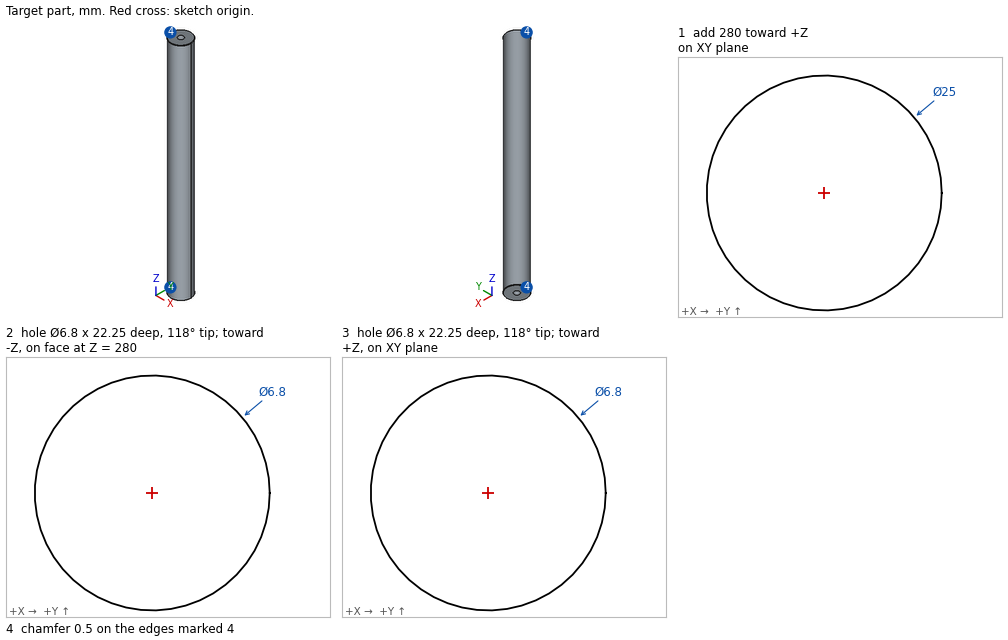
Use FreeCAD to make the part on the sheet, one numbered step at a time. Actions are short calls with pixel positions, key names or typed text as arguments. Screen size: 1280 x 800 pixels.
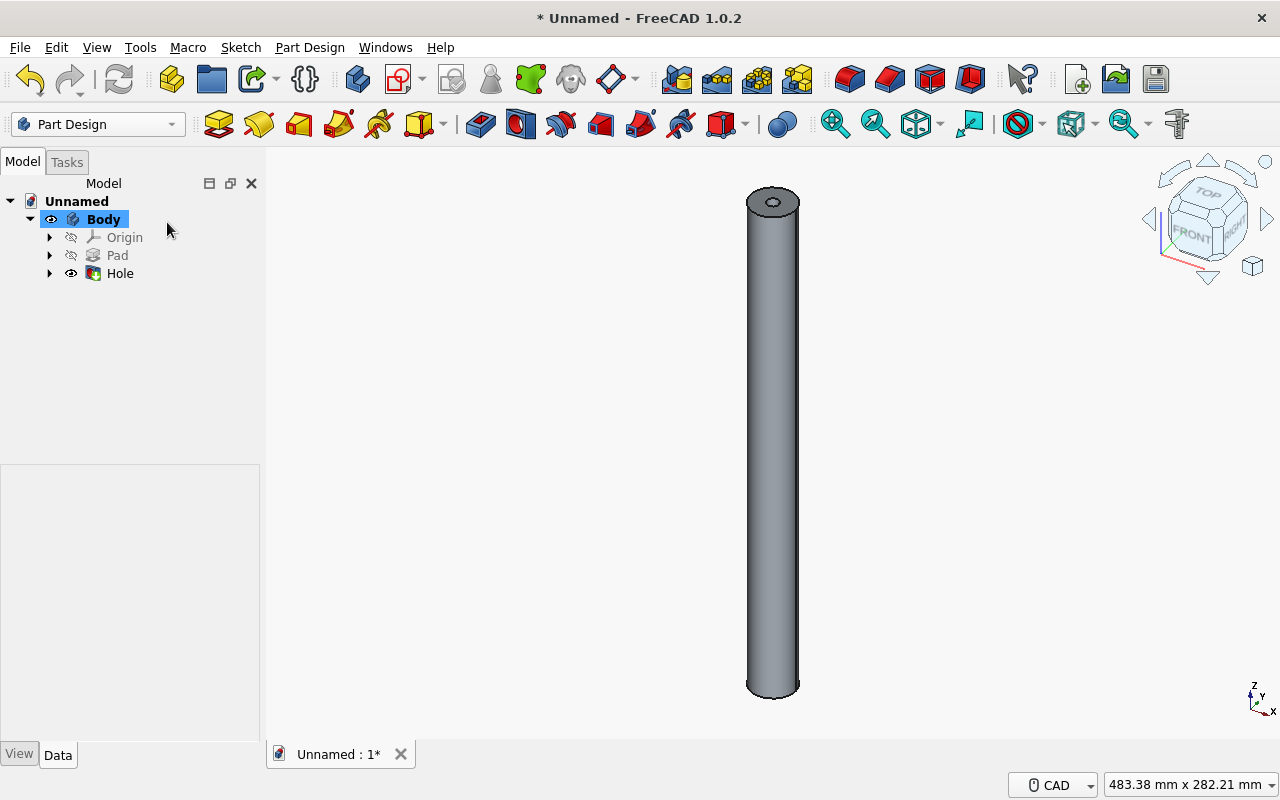
click(398, 80)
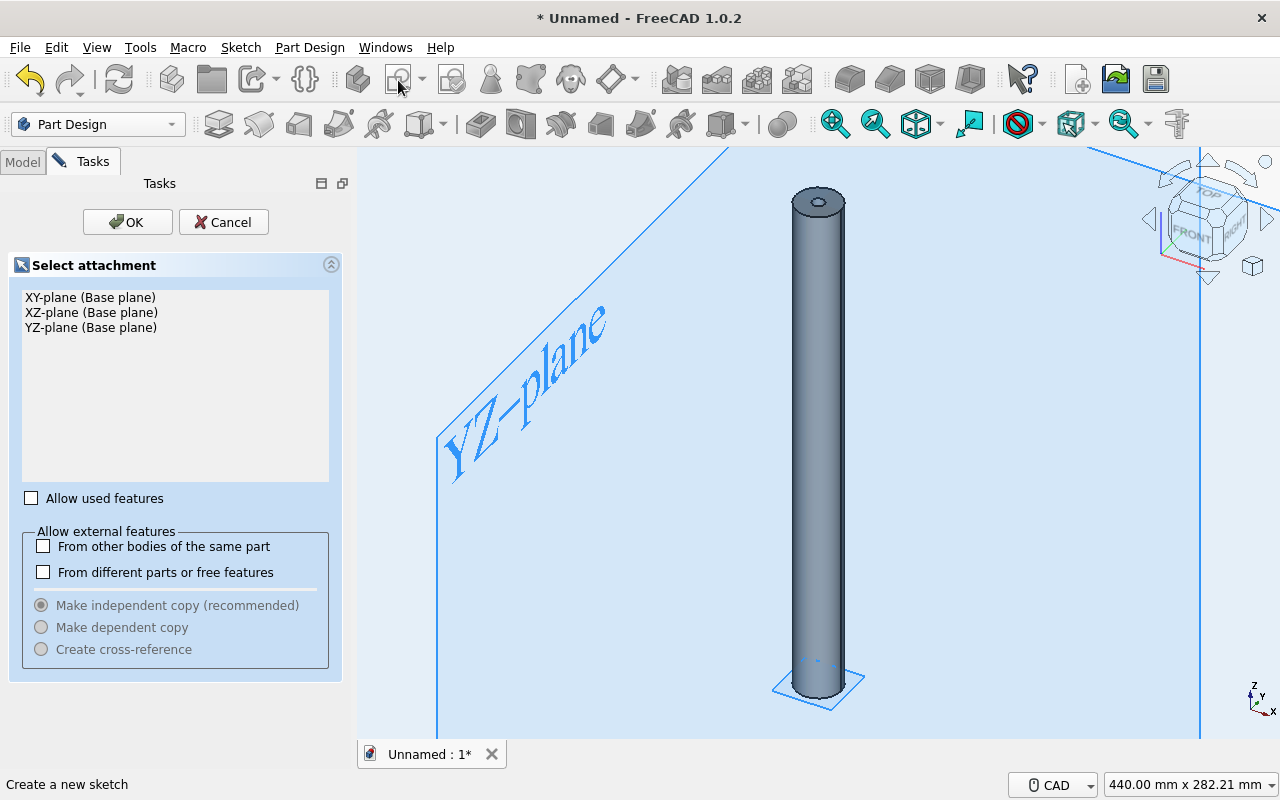
click(82, 298)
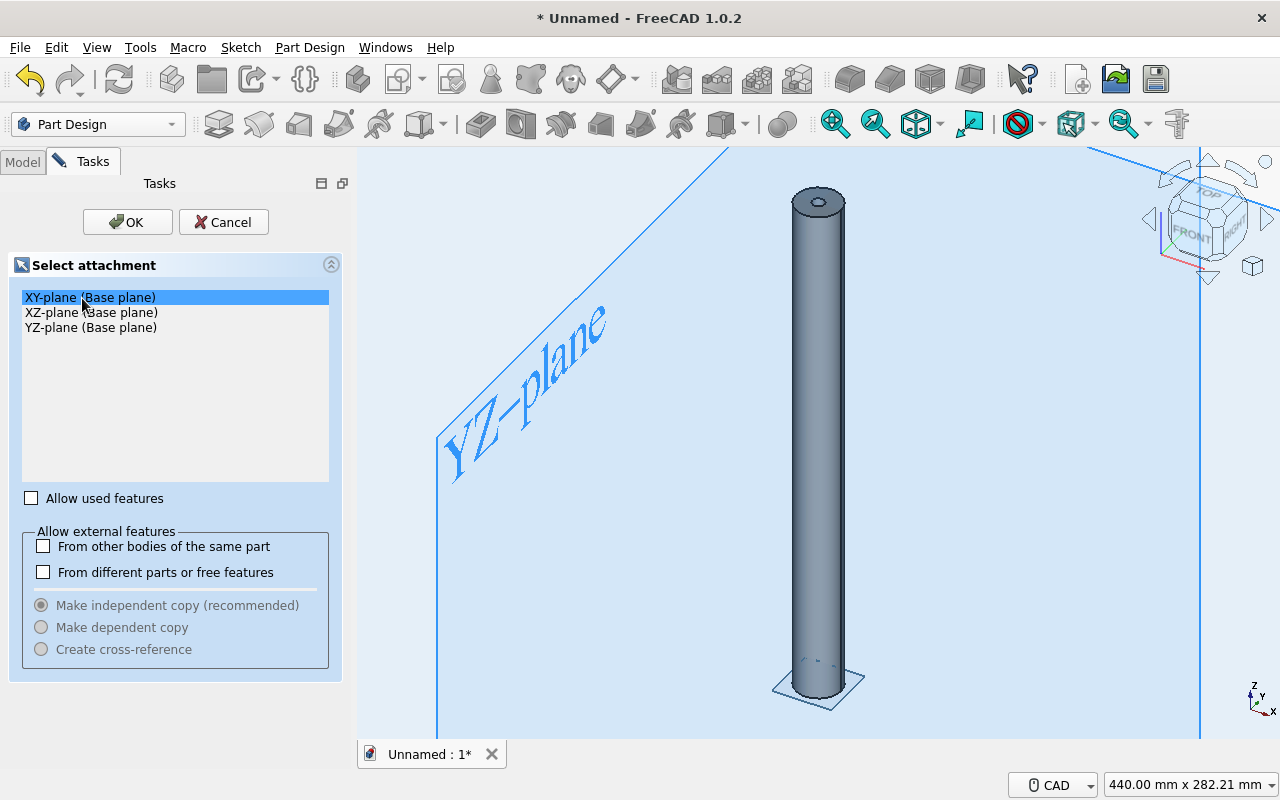
click(128, 222)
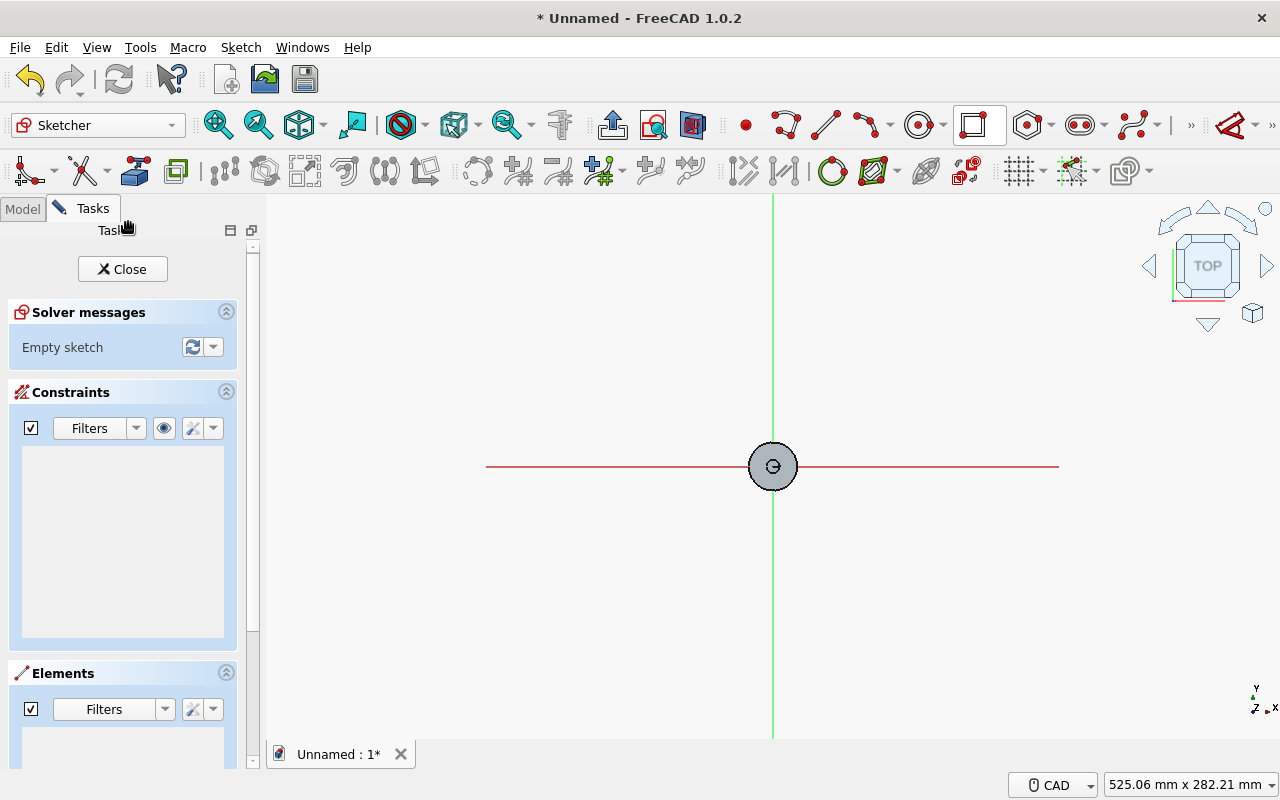
click(694, 126)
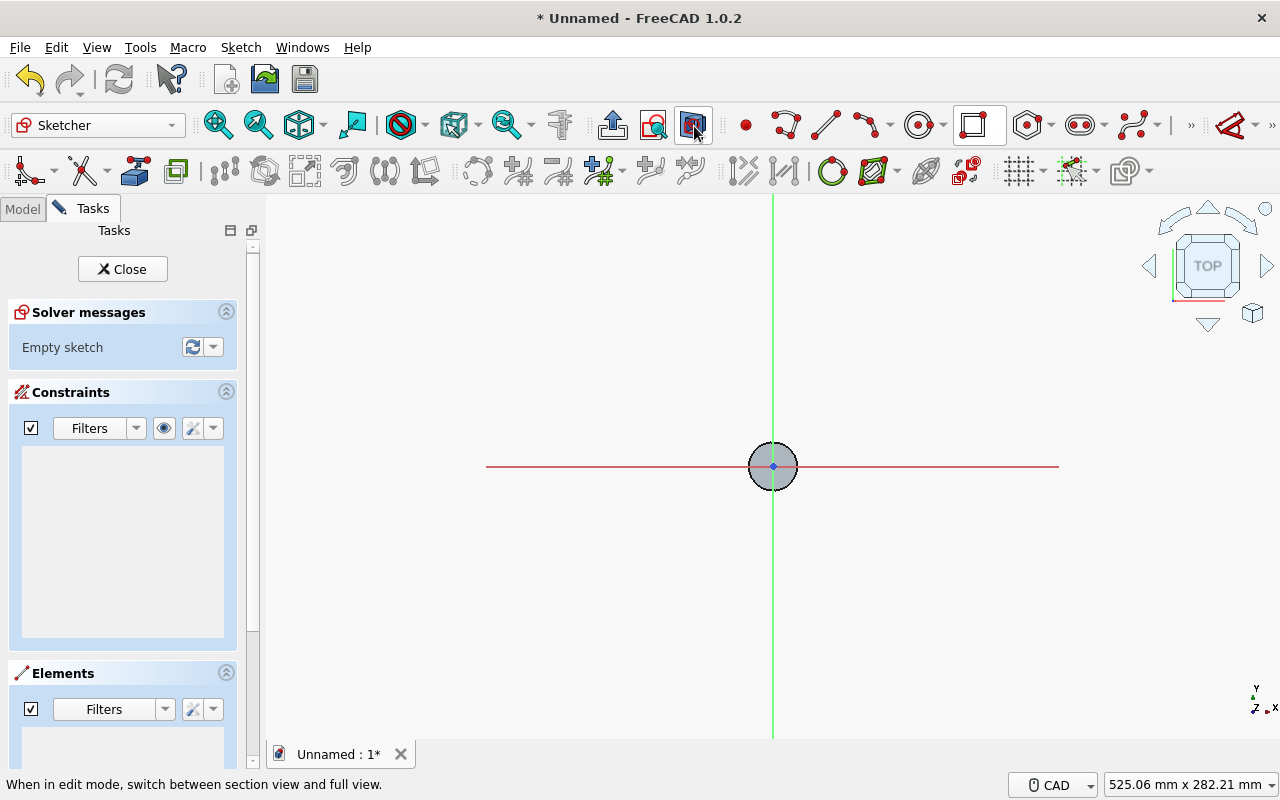
scroll(777, 466, up, 15)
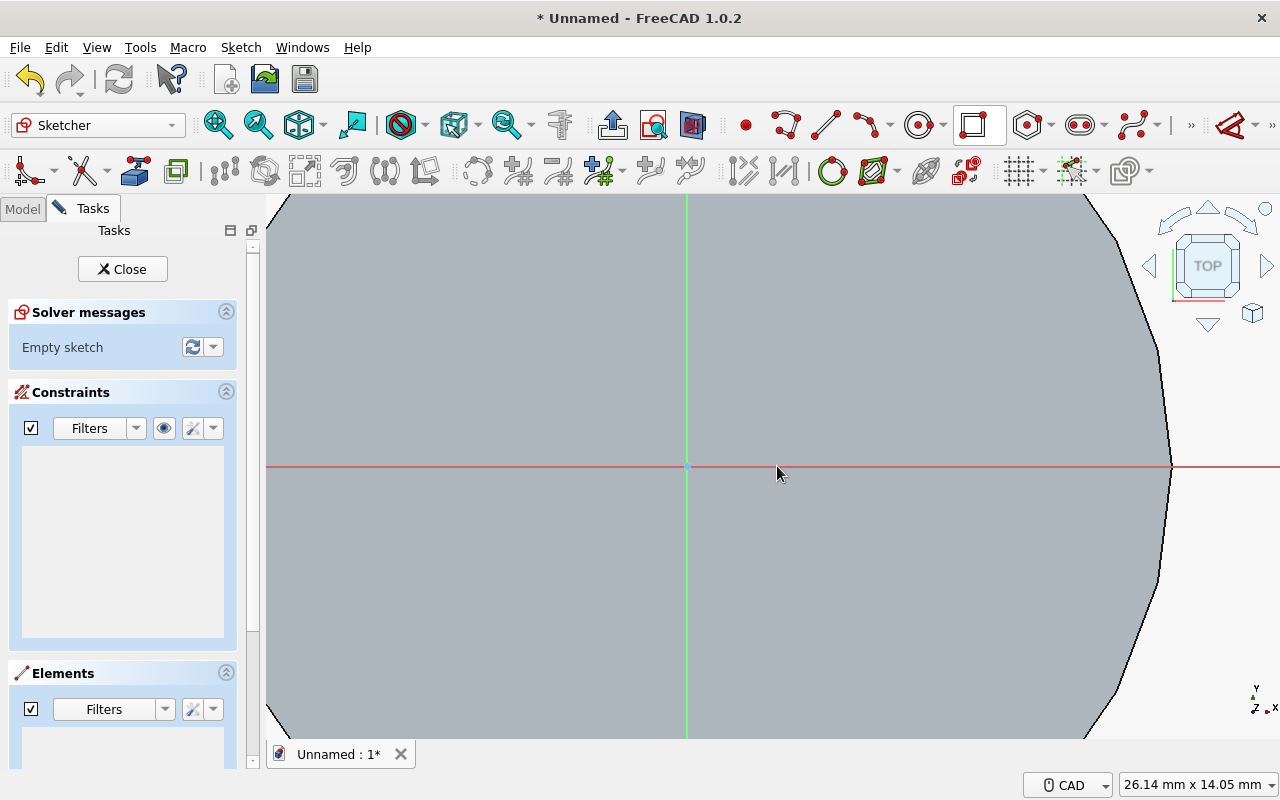
click(920, 126)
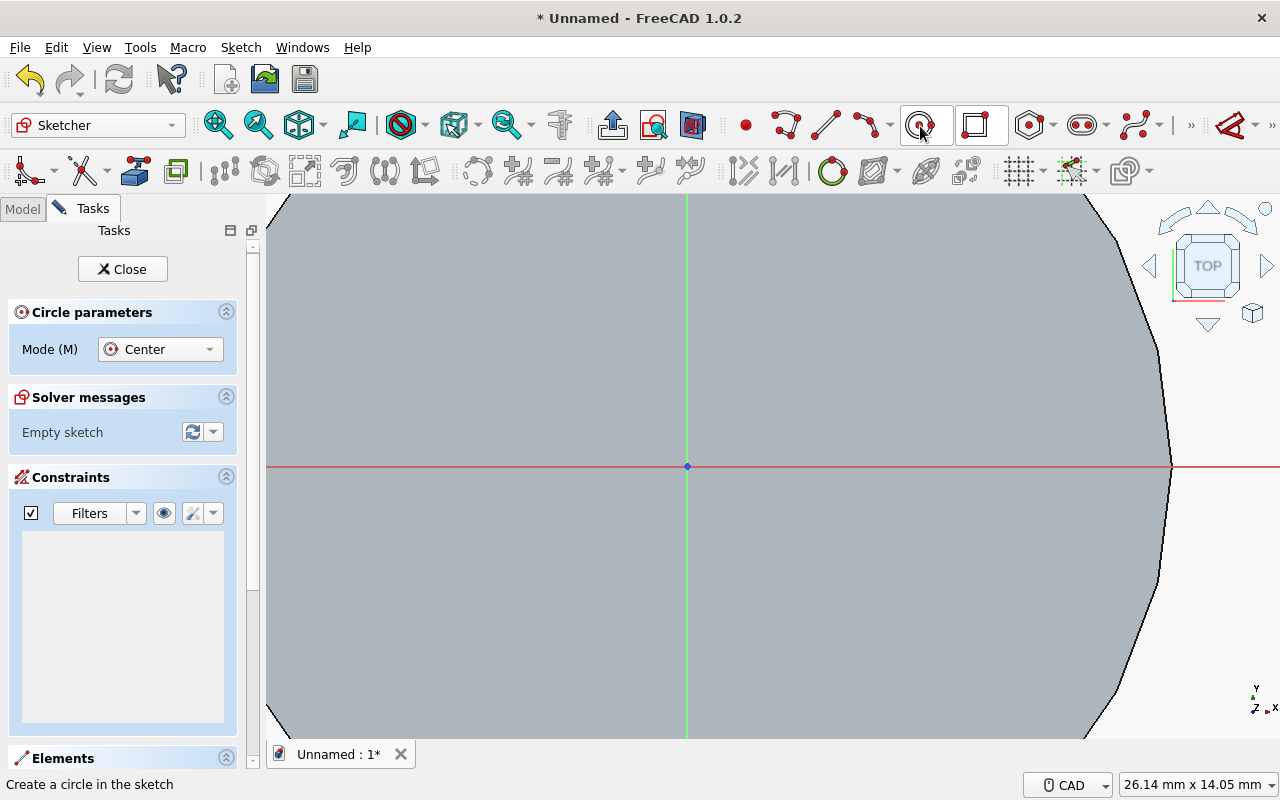
click(687, 466)
click(780, 373)
key(Escape)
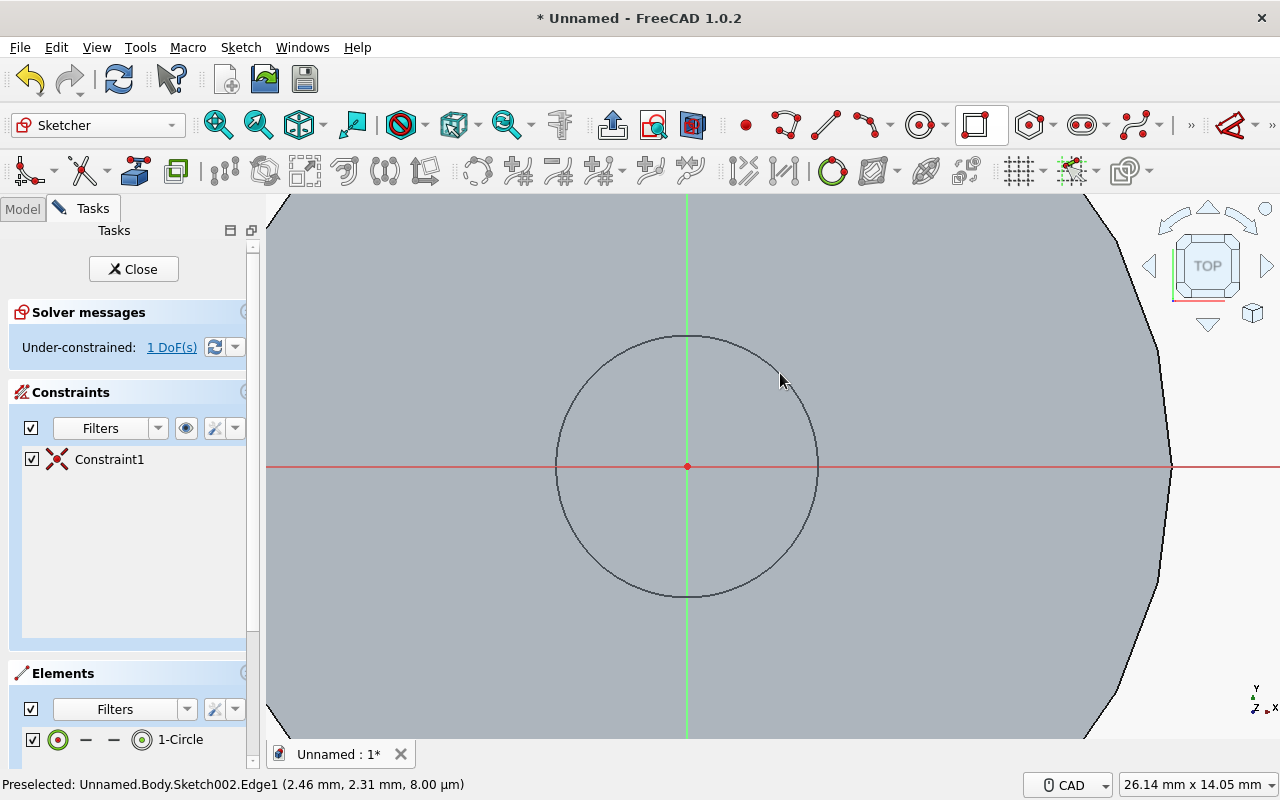
click(1230, 126)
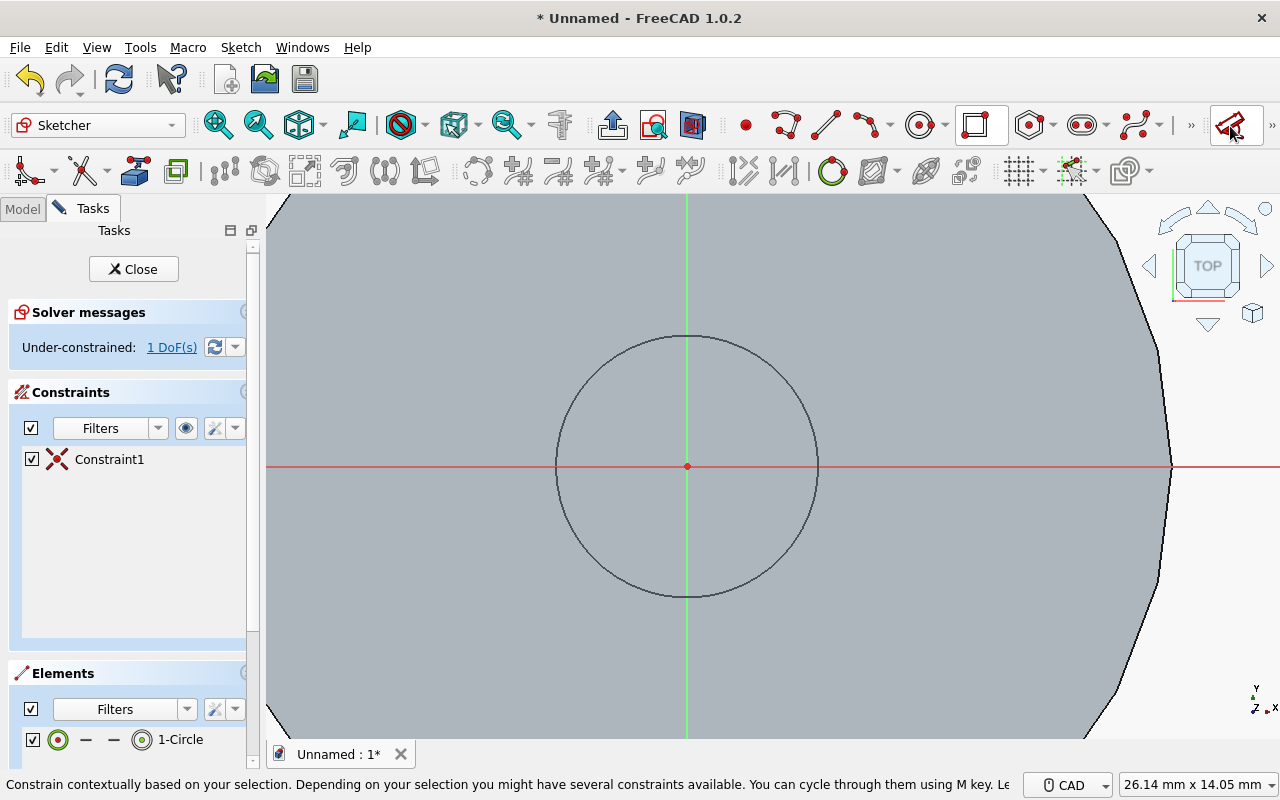
click(779, 373)
click(801, 350)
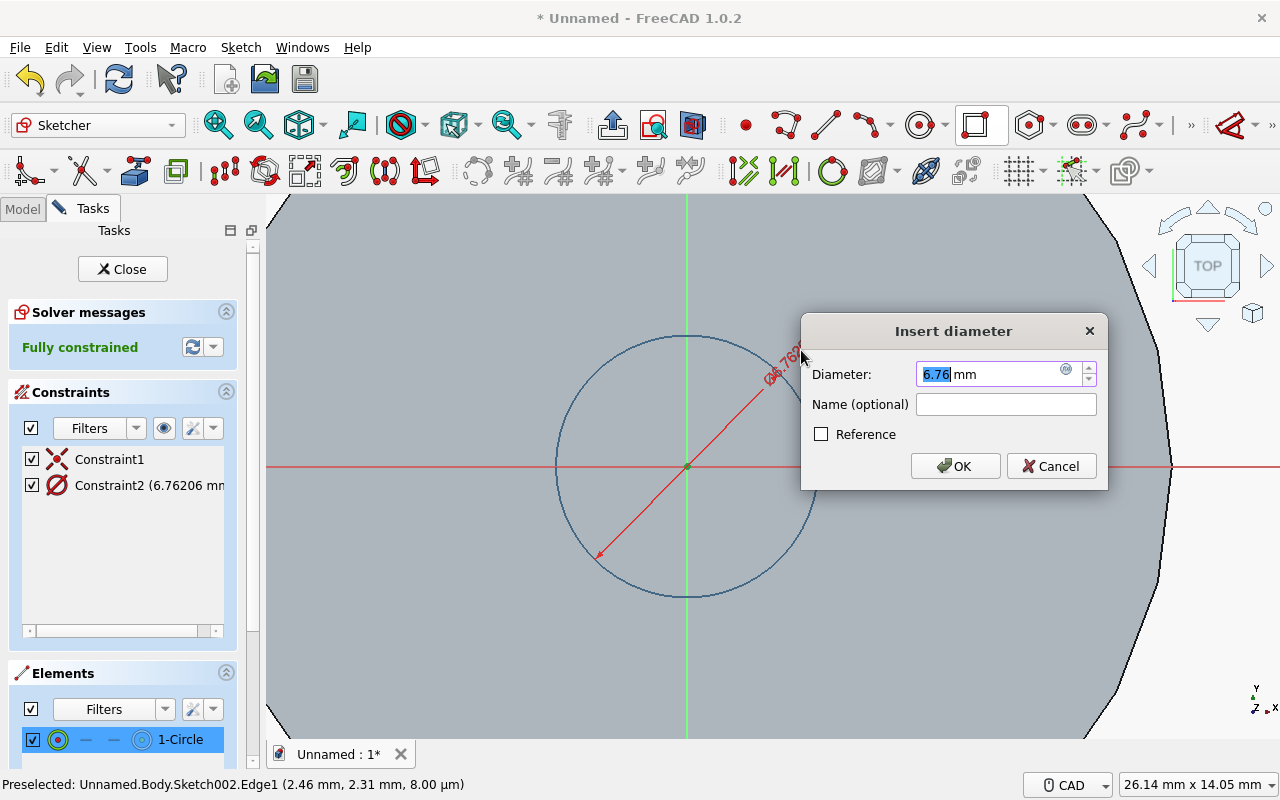
text(6.8)
key(Return)
key(Escape)